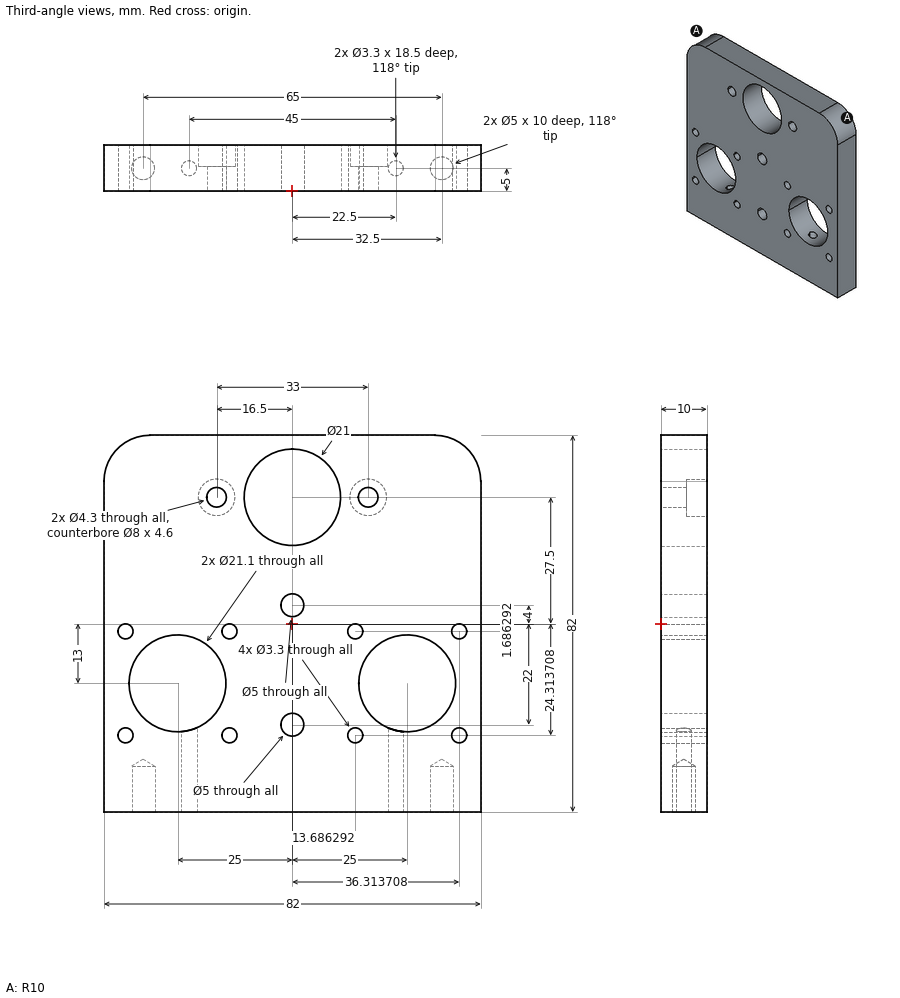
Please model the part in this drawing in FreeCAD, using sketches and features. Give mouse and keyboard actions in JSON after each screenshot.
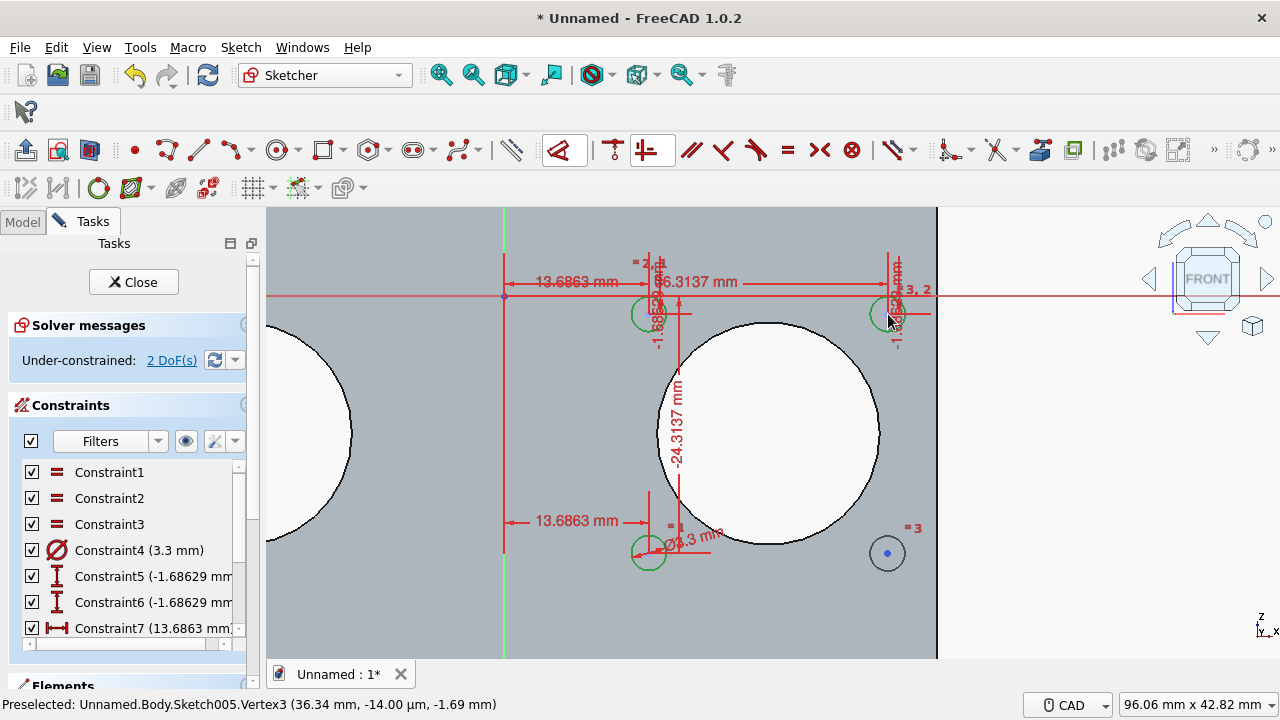
{"action": "left_click", "coordinate": [888, 554]}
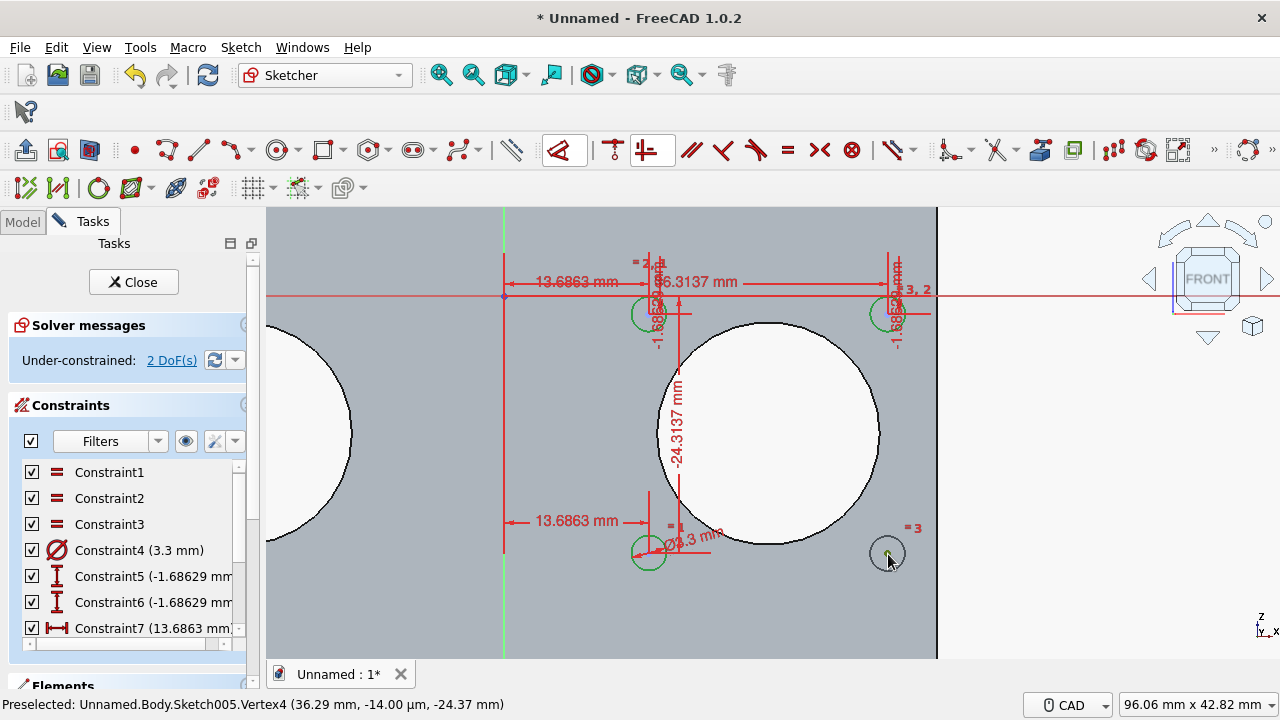
{"action": "key", "text": "l"}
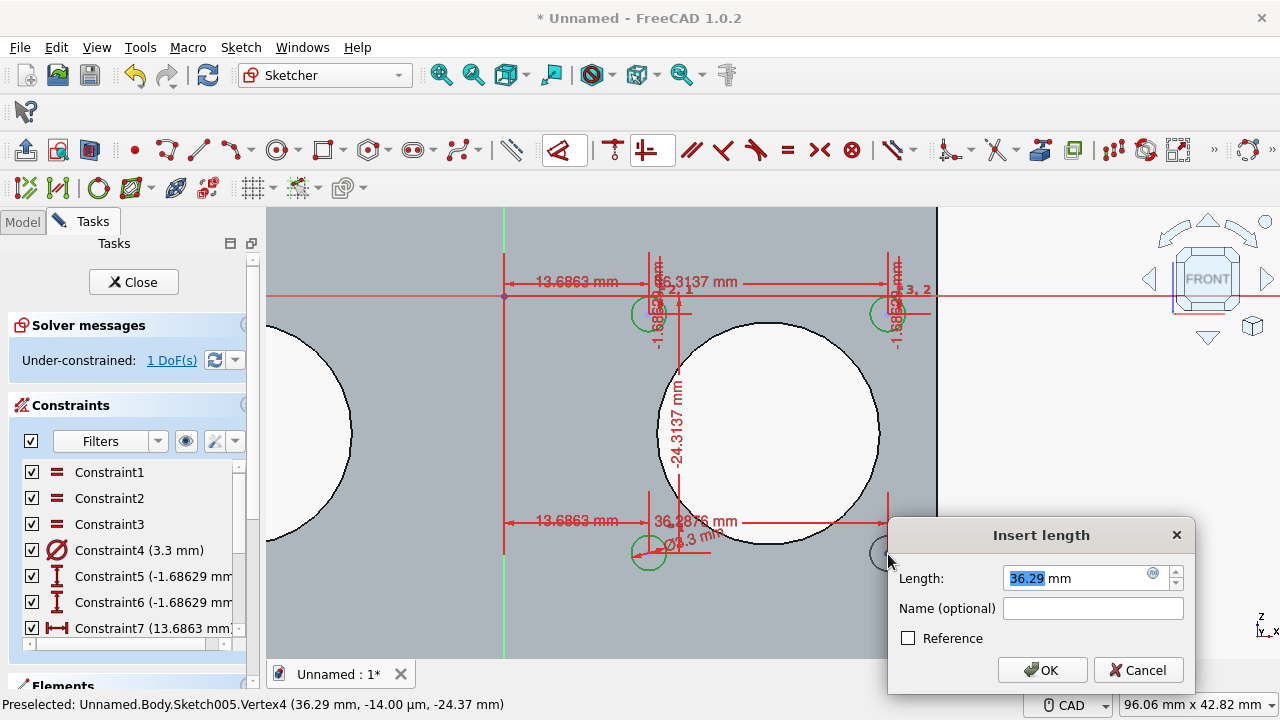
{"action": "type", "text": "36.313708"}
{"action": "key", "text": "Return"}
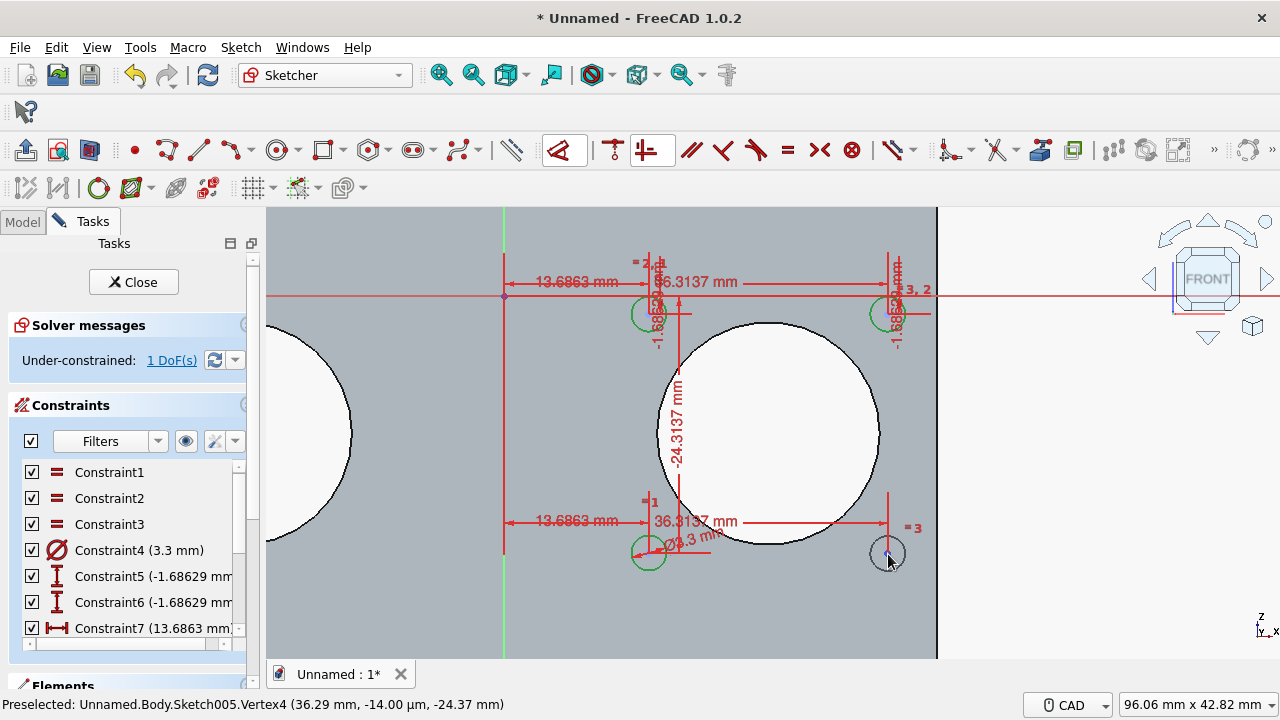
{"action": "left_click", "coordinate": [888, 554]}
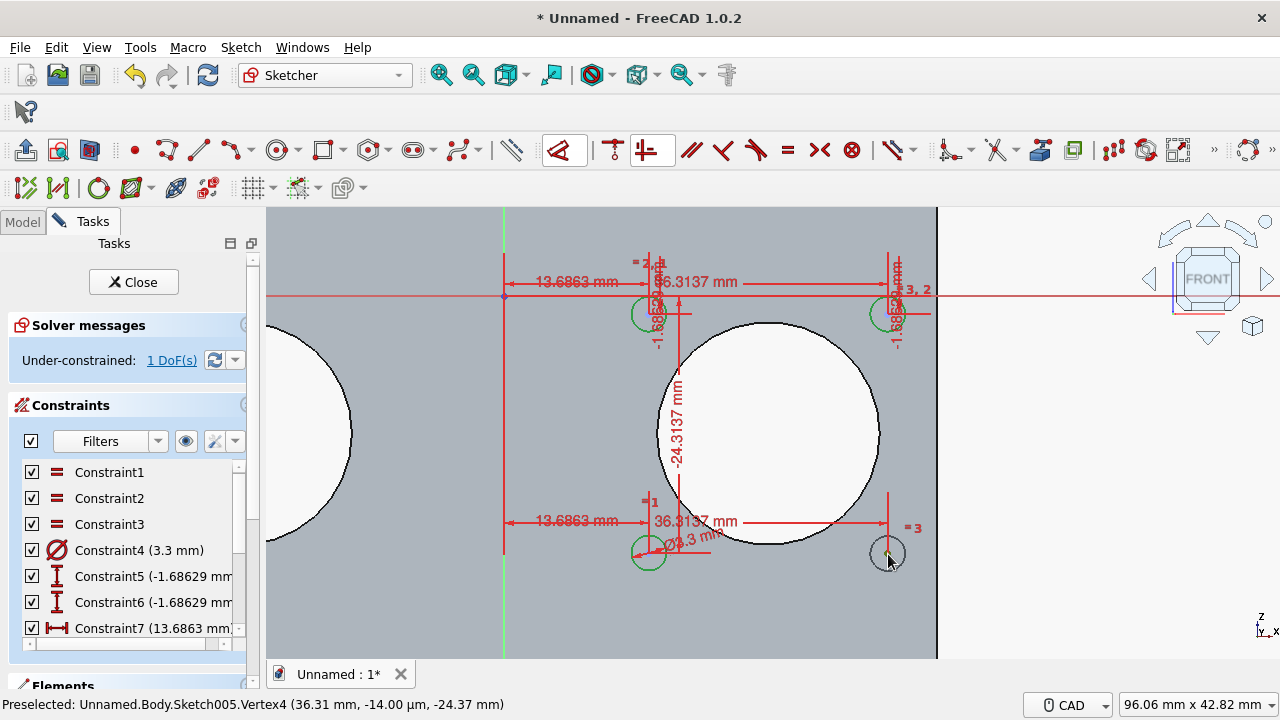
{"action": "key", "text": "i"}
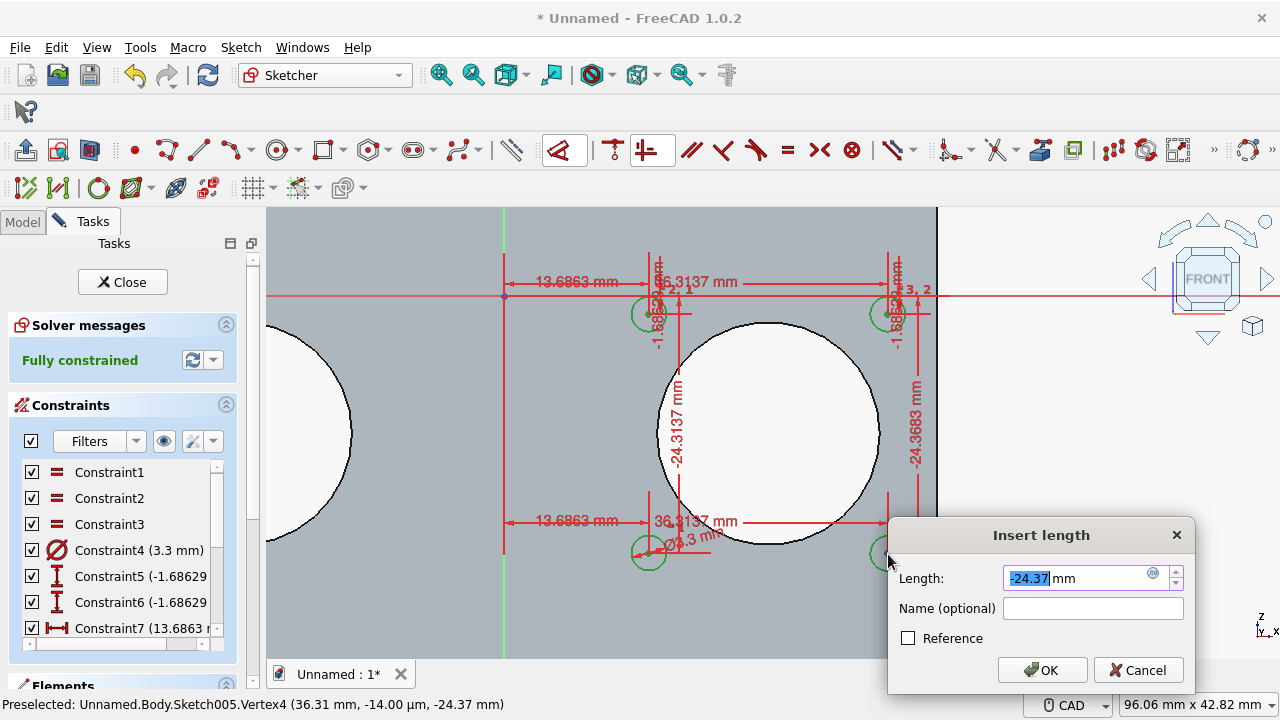
{"action": "type", "text": "-24.313708"}
{"action": "key", "text": "Return"}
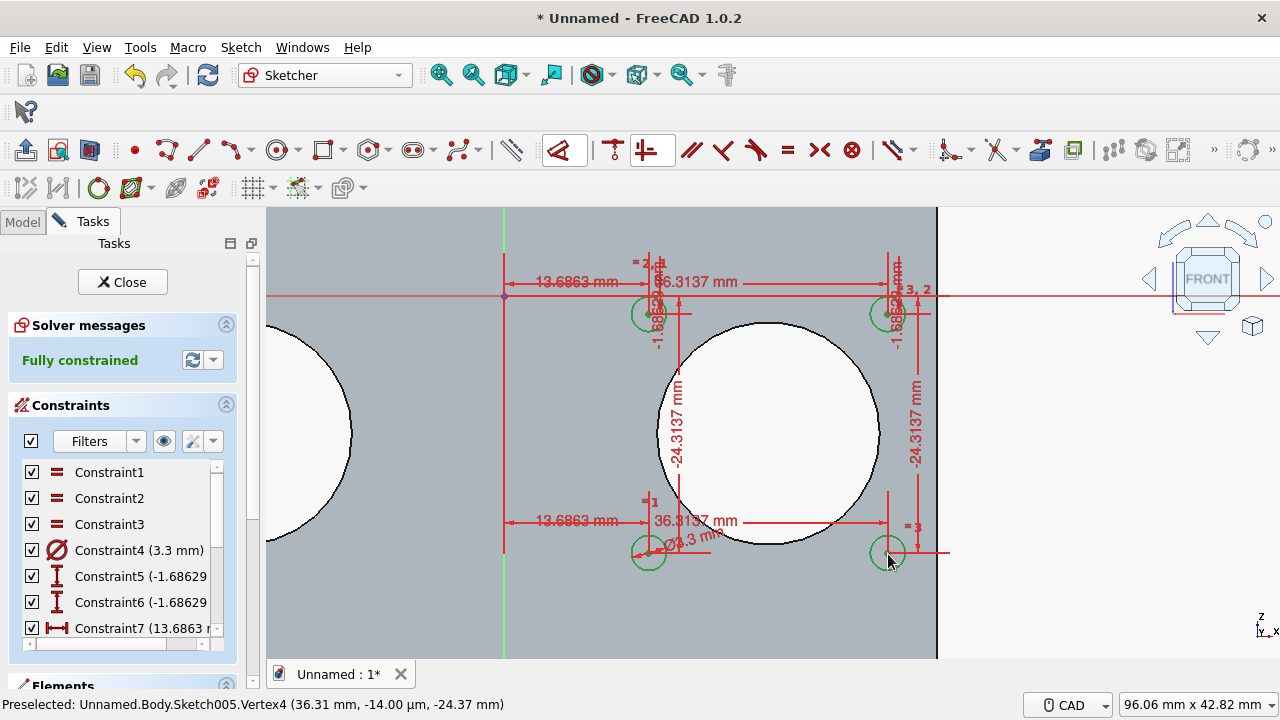
{"action": "left_click", "coordinate": [123, 282]}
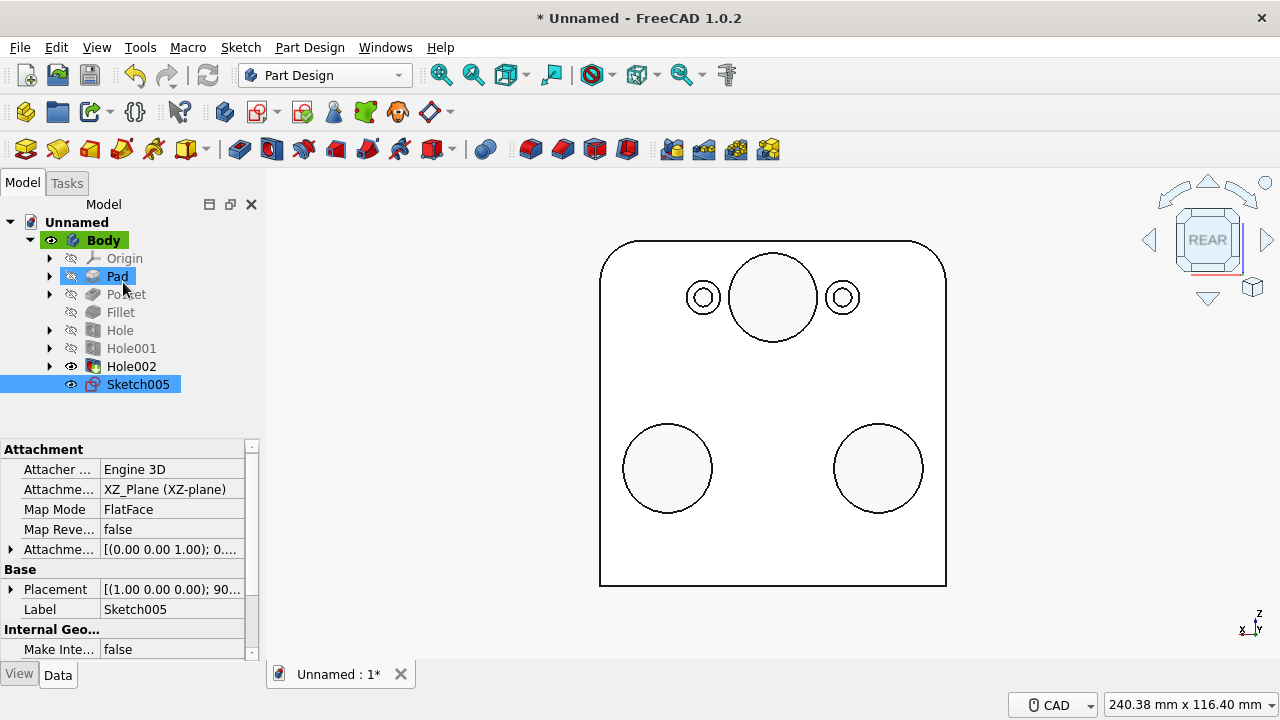
{"action": "left_click", "coordinate": [272, 150]}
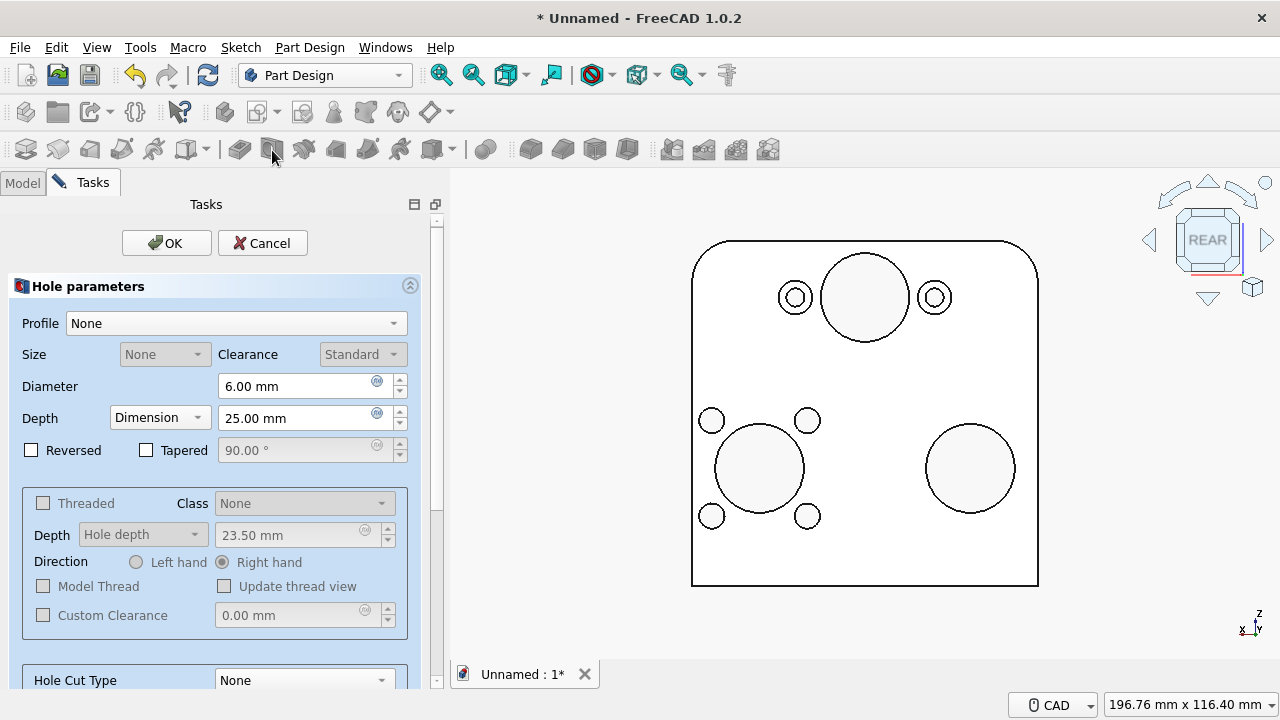
{"action": "triple_click", "coordinate": [305, 386]}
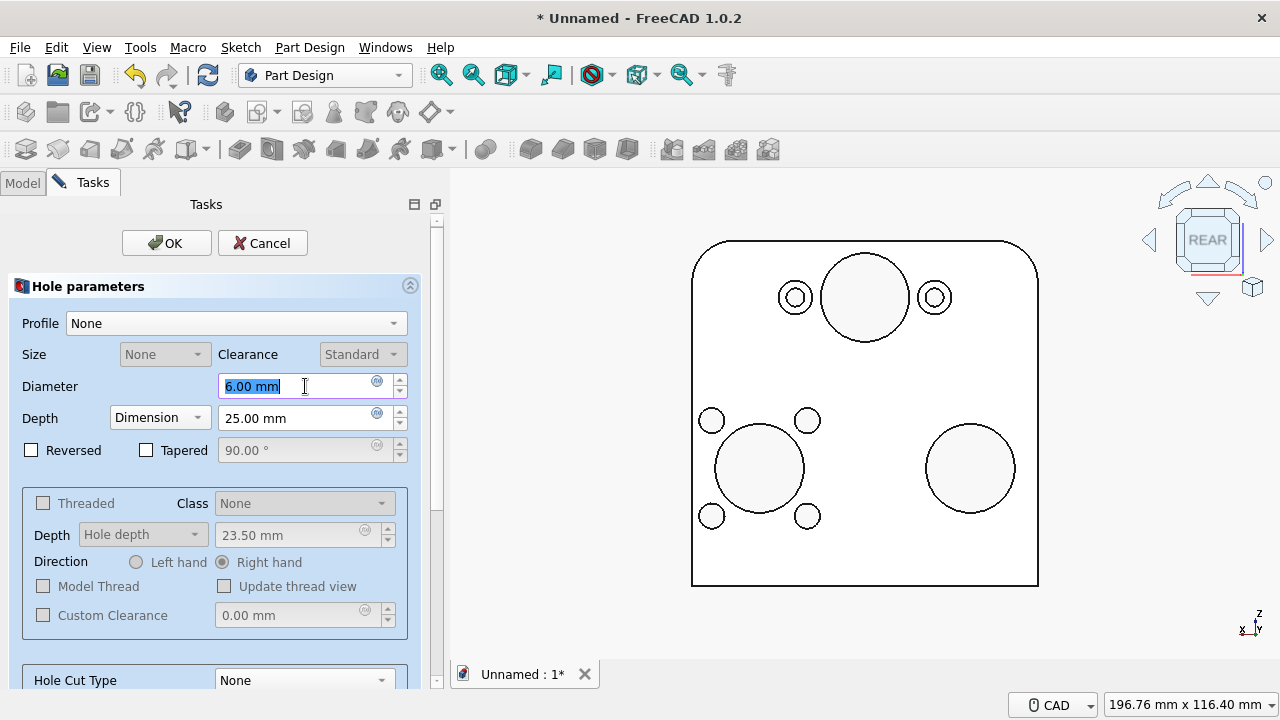
{"action": "type", "text": "3.3"}
{"action": "key", "text": "Tab"}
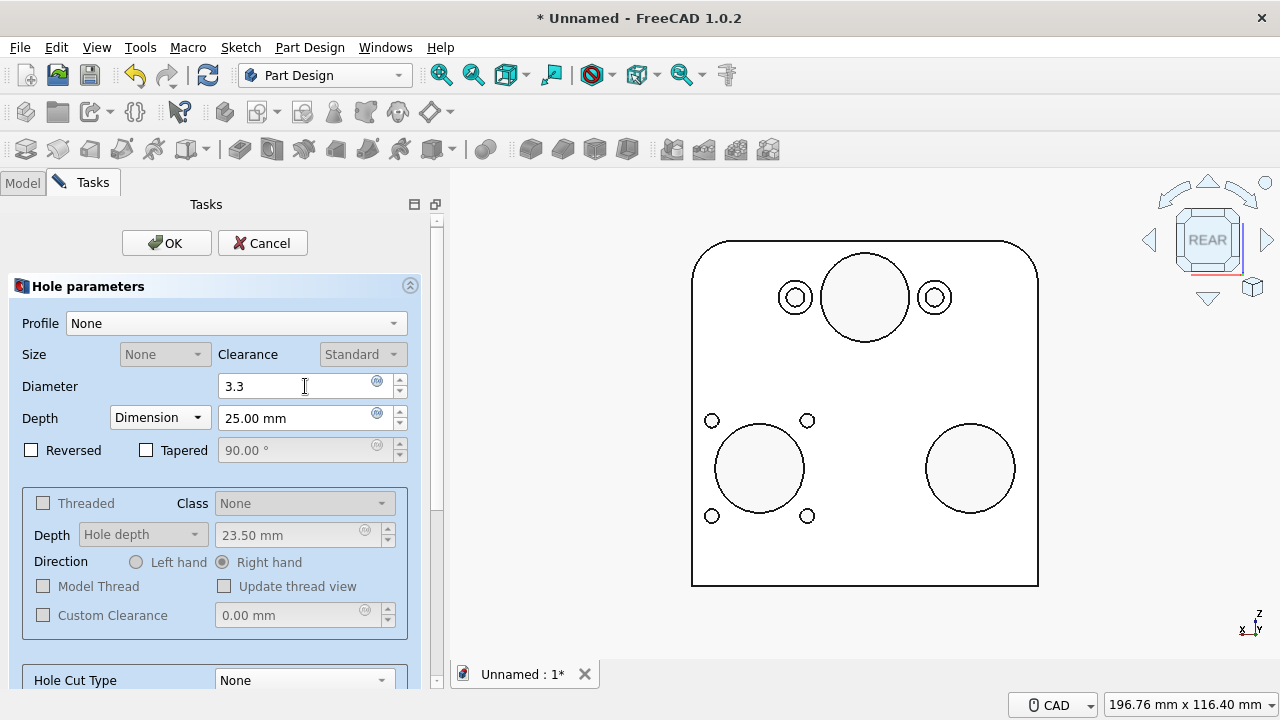
{"action": "left_click", "coordinate": [161, 418]}